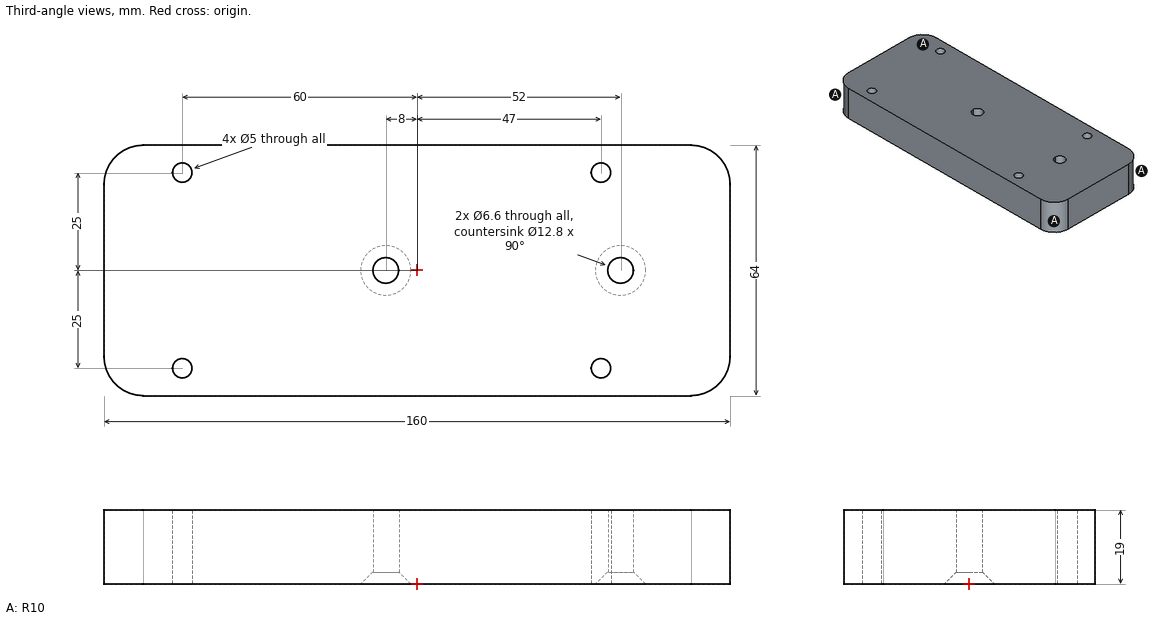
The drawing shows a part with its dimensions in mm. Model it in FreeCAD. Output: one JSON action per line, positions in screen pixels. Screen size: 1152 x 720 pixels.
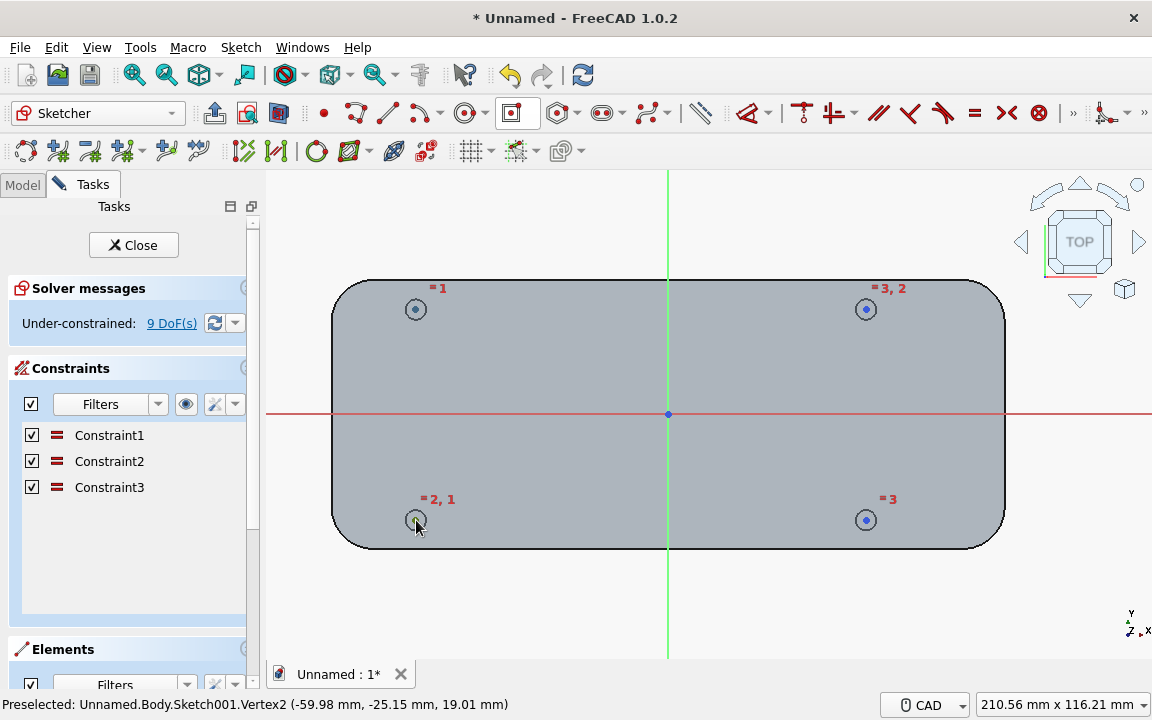
{"action": "key", "text": "v"}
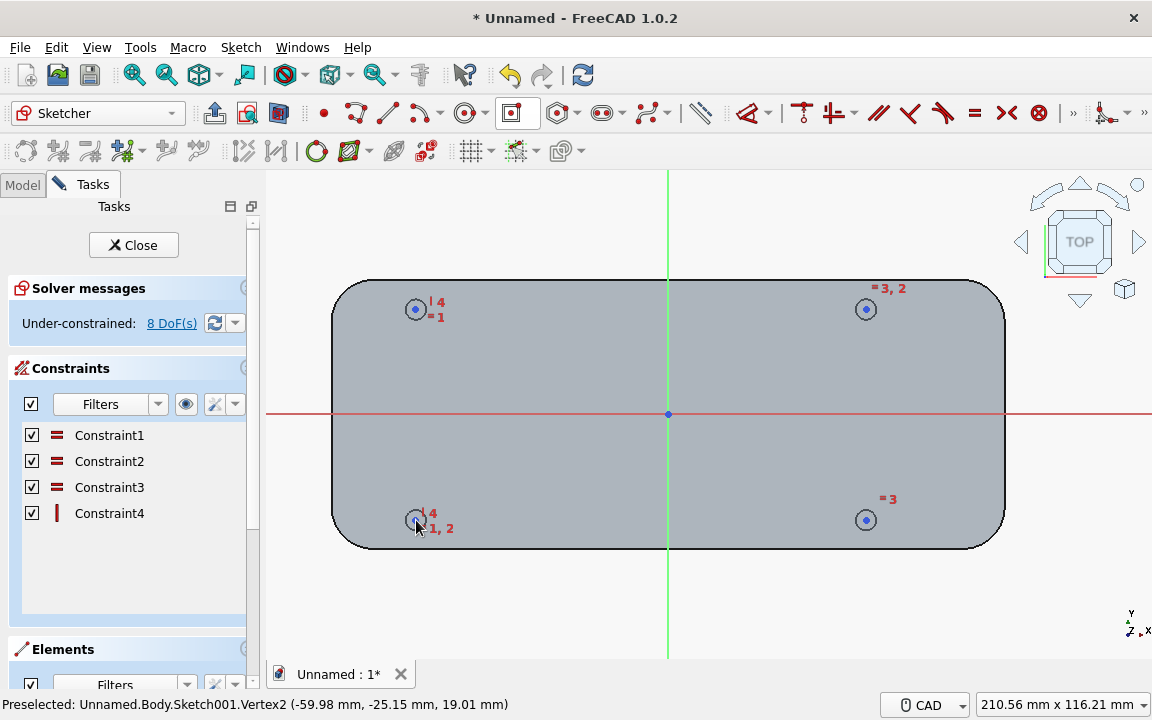
{"action": "left_click", "coordinate": [416, 310]}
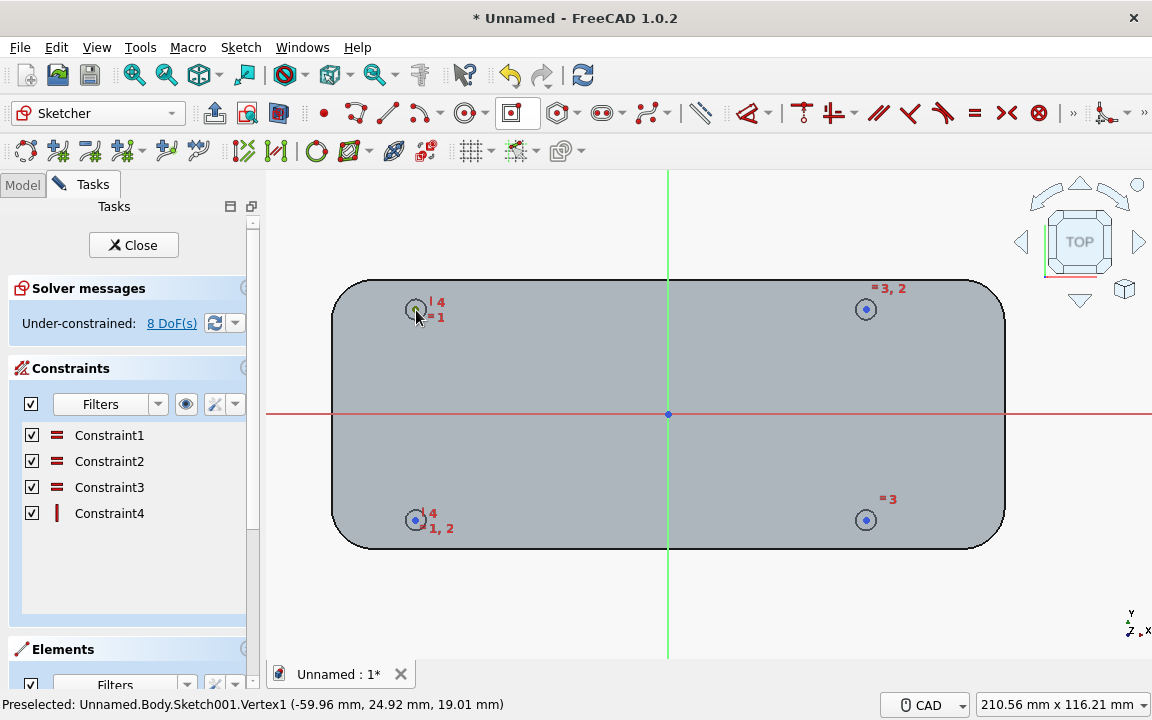
{"action": "left_click", "coordinate": [866, 309]}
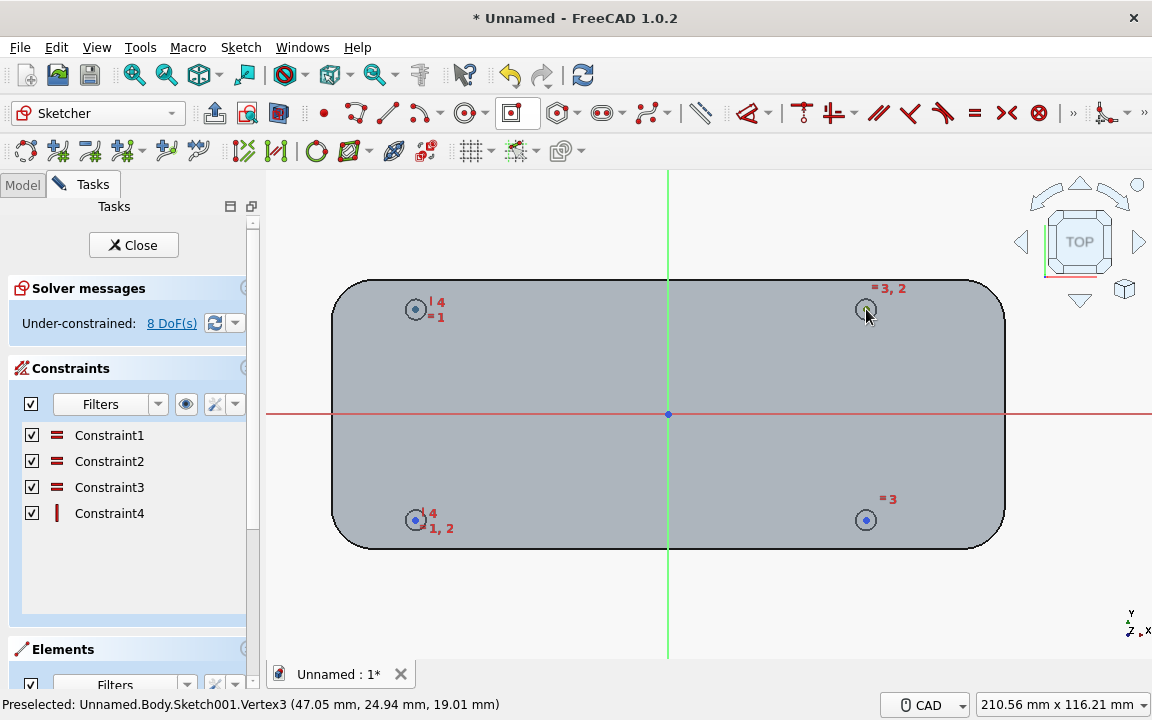
{"action": "left_click", "coordinate": [856, 114]}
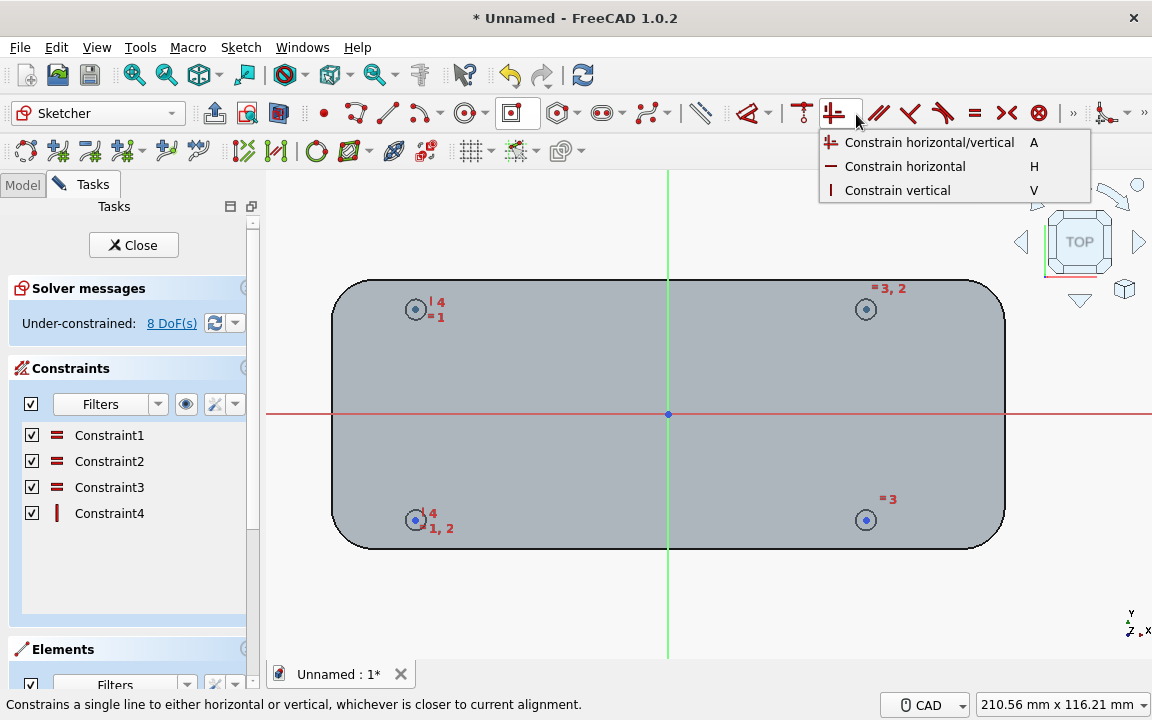
{"action": "left_click", "coordinate": [955, 166]}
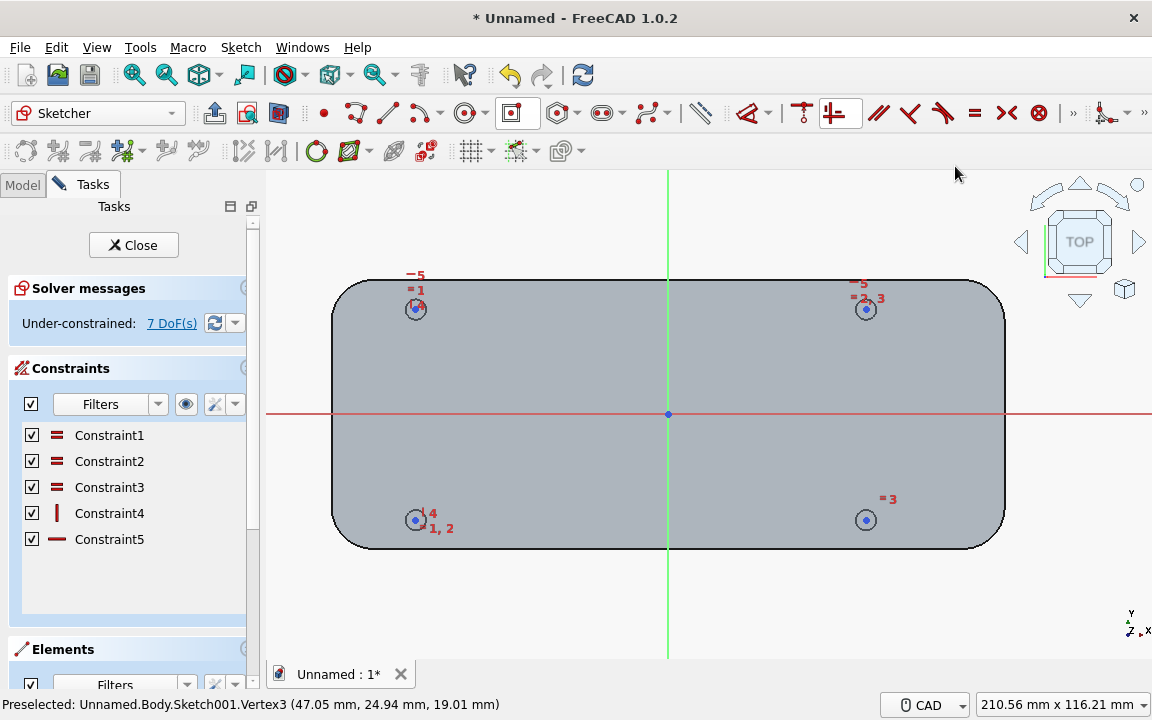
{"action": "left_click", "coordinate": [866, 310]}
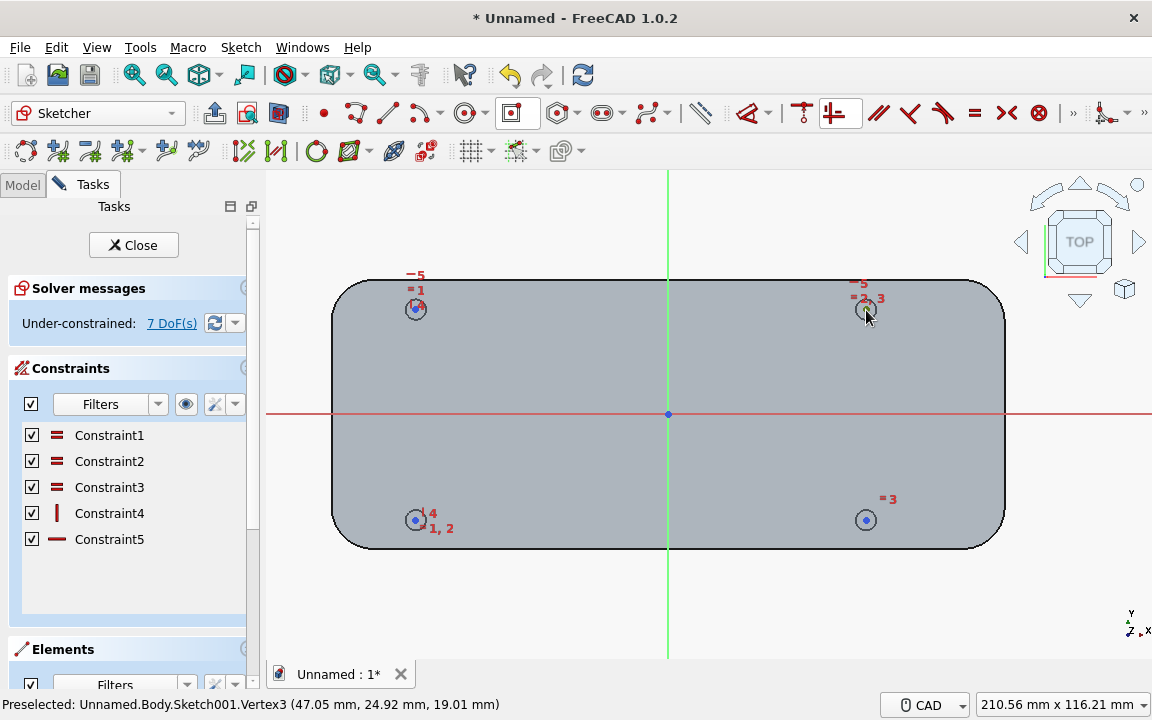
{"action": "left_click", "coordinate": [866, 520]}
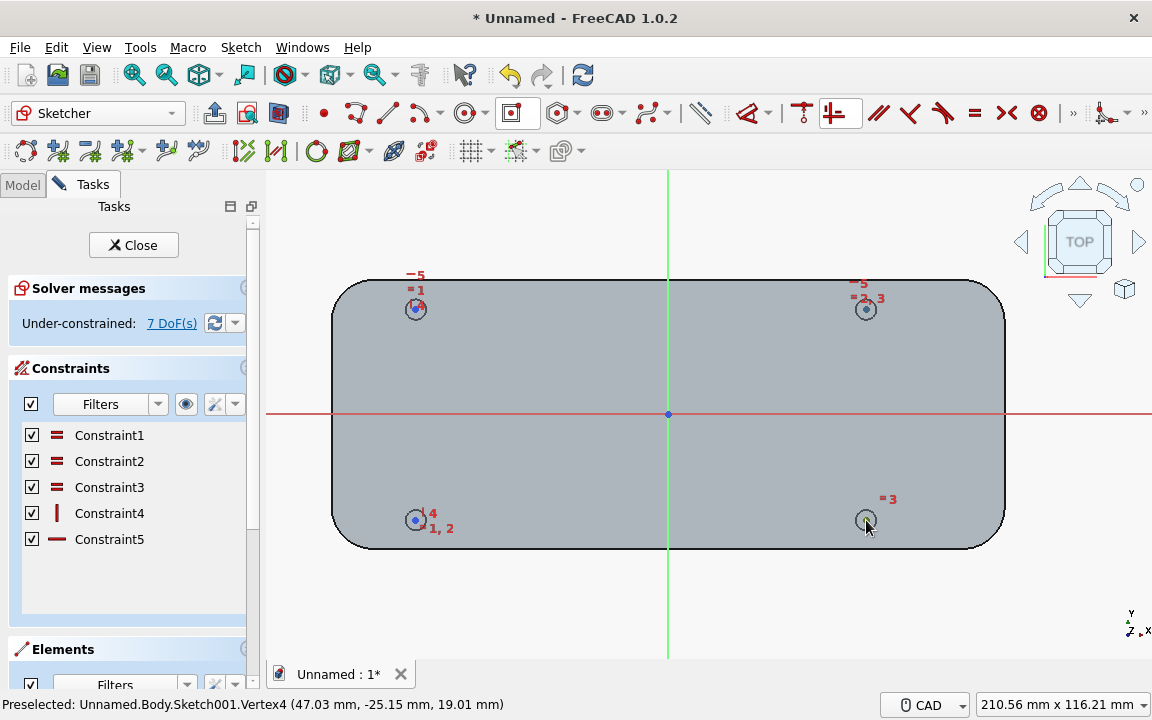
{"action": "key", "text": "v"}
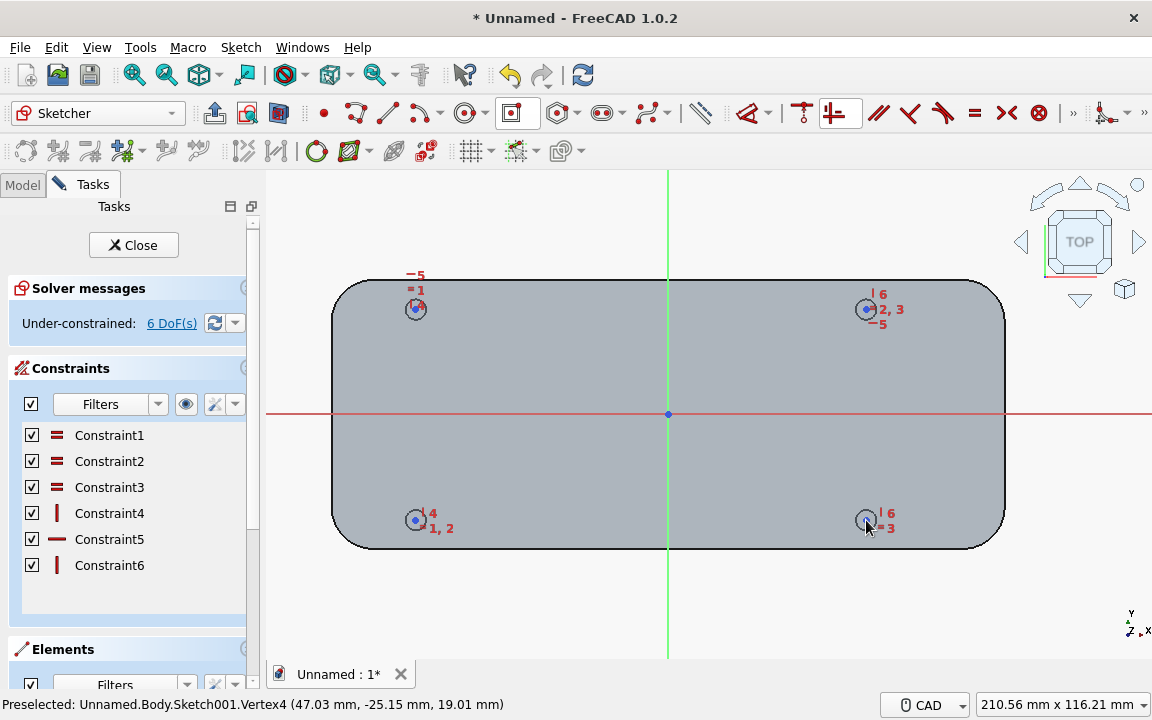
{"action": "left_click", "coordinate": [416, 520]}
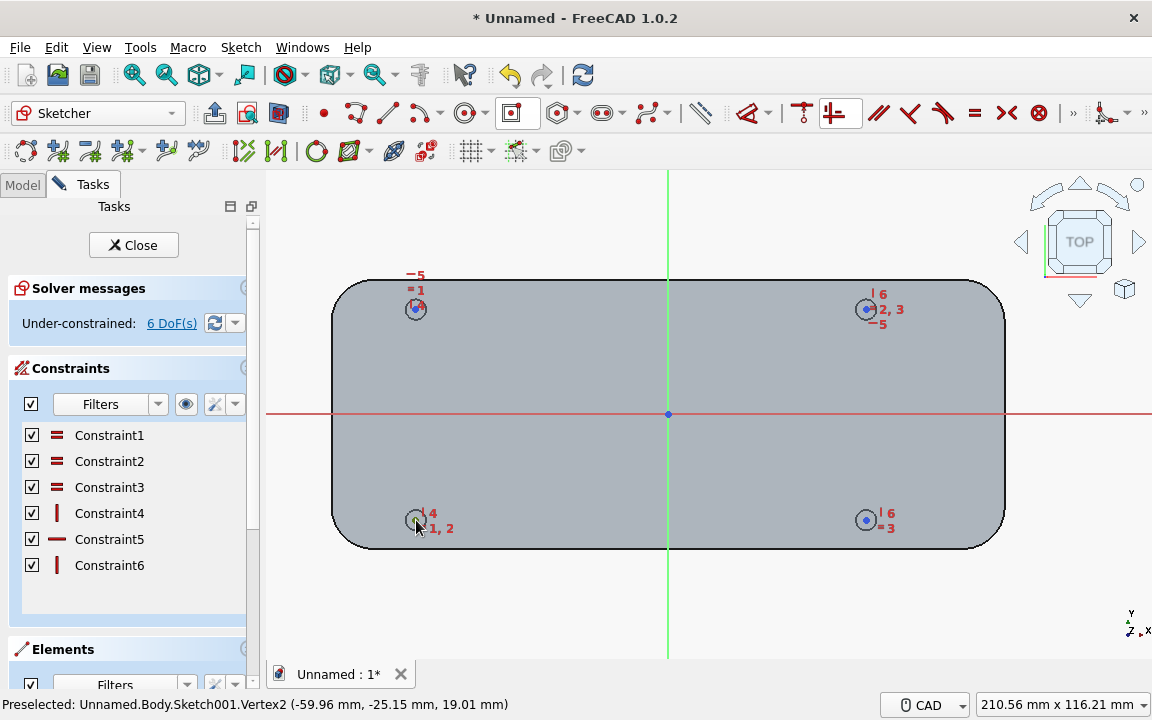
{"action": "left_click", "coordinate": [866, 520]}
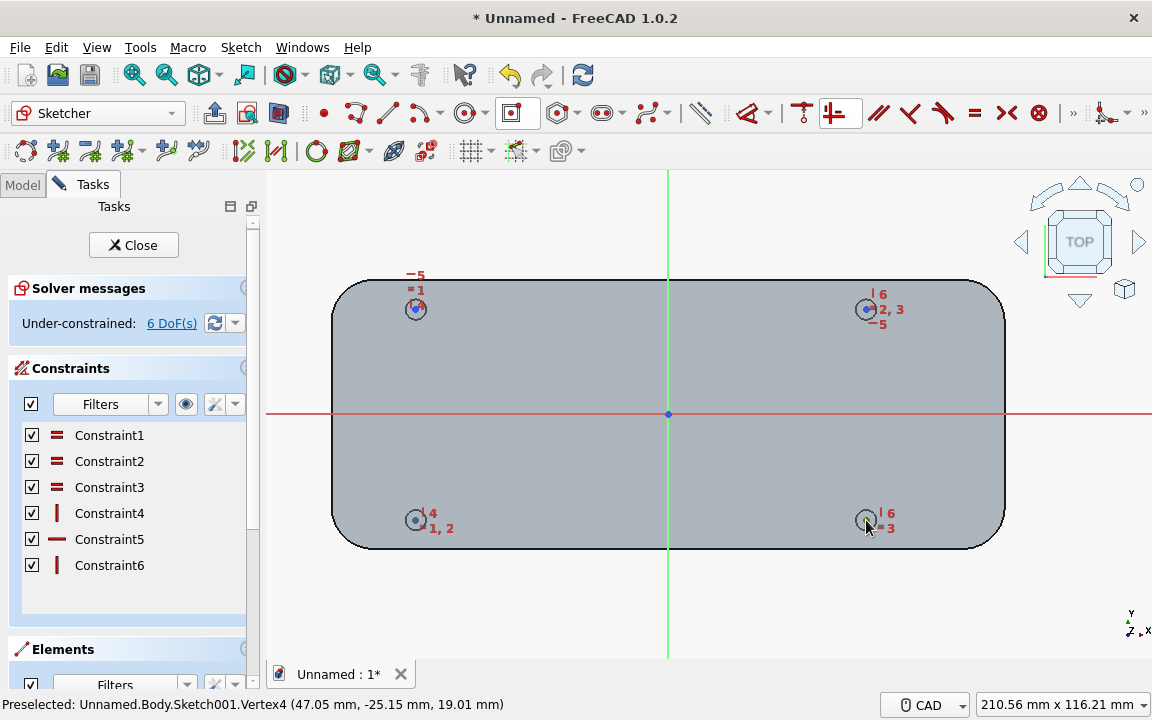
{"action": "left_click", "coordinate": [856, 114]}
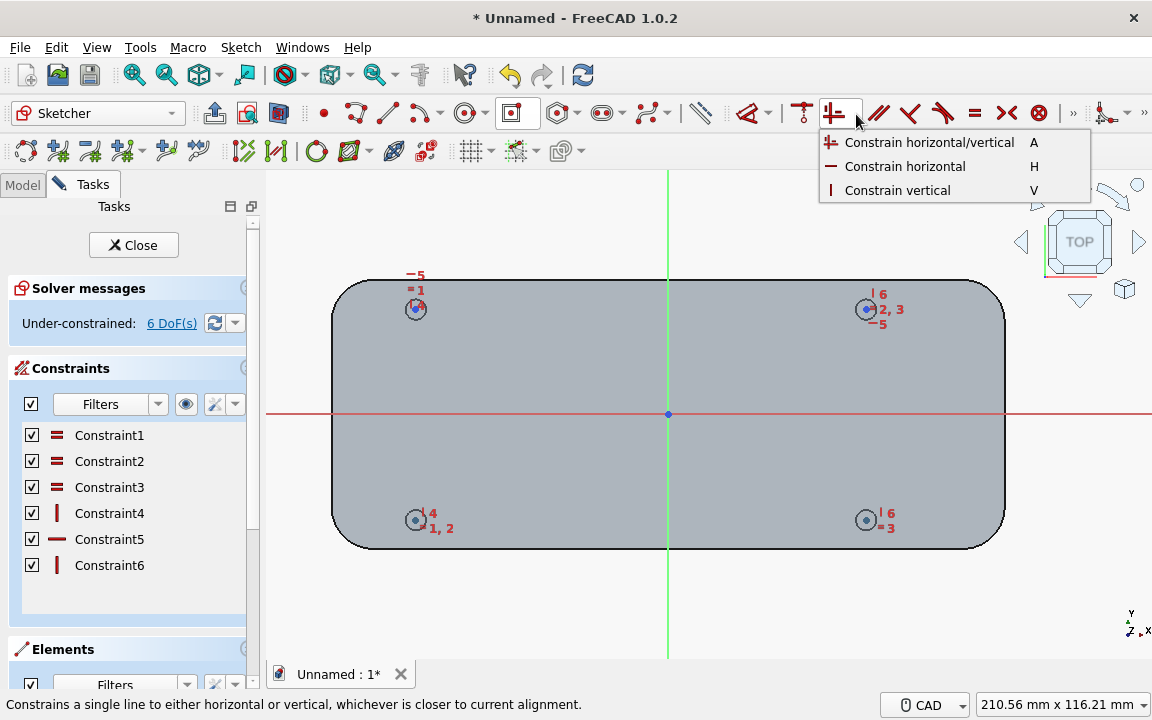
{"action": "left_click", "coordinate": [955, 166]}